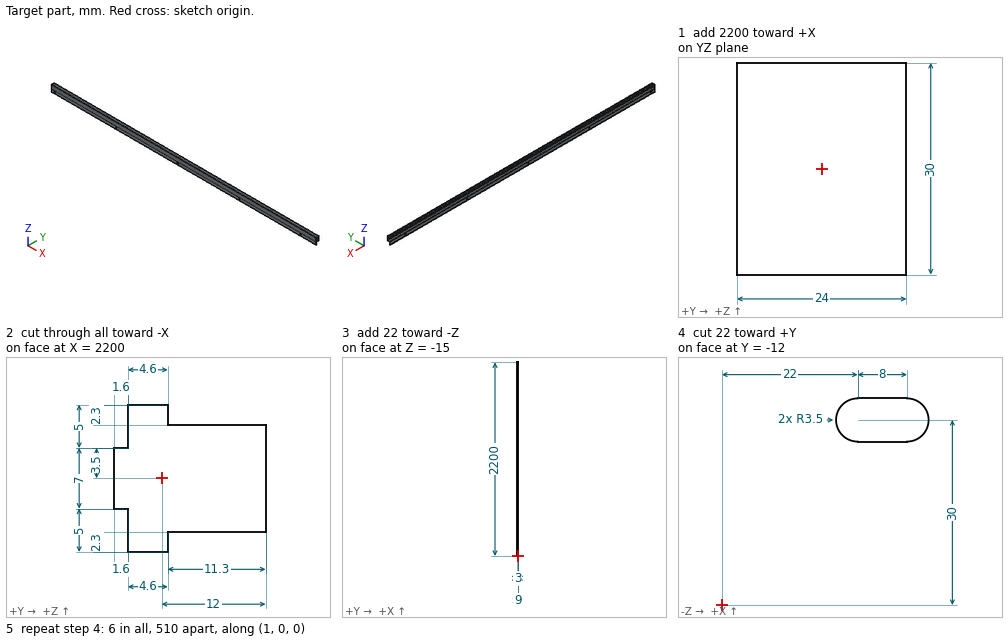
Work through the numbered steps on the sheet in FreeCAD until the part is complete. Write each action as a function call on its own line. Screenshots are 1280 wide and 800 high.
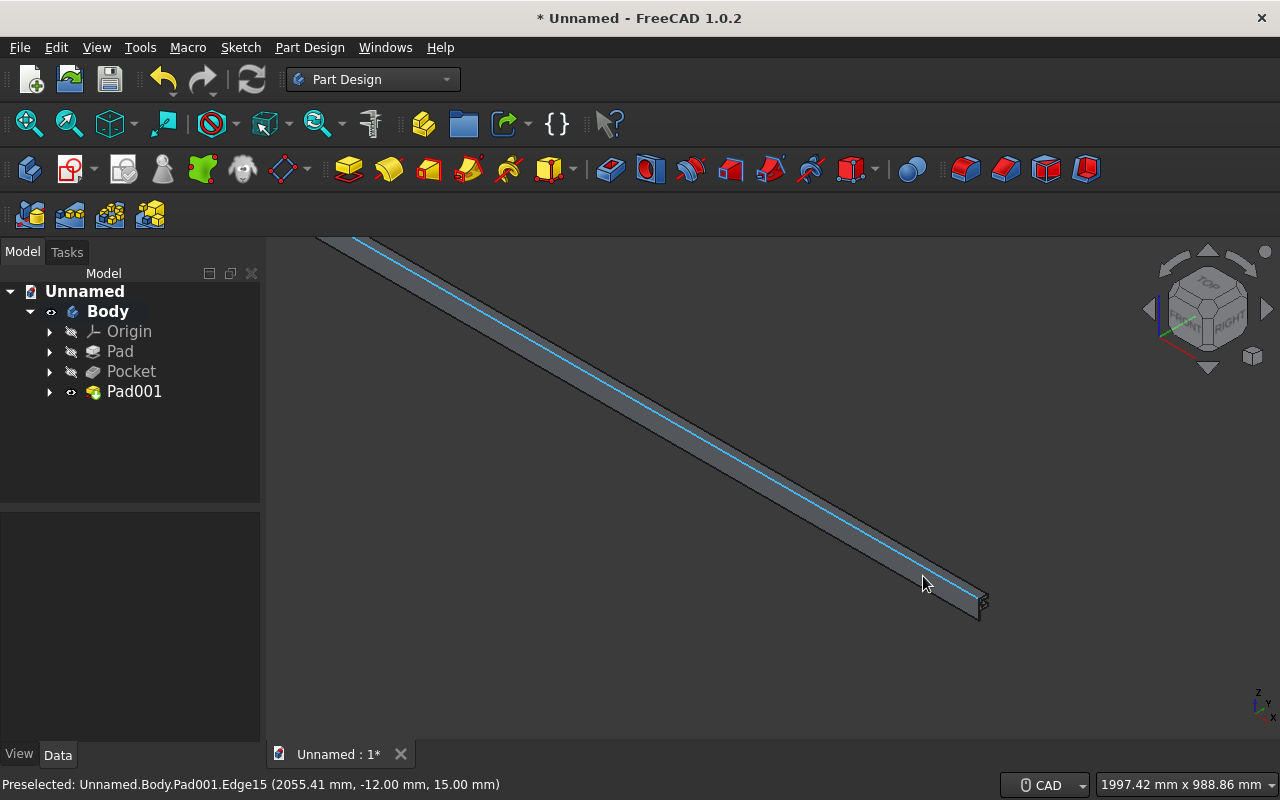
key(v)
key(f)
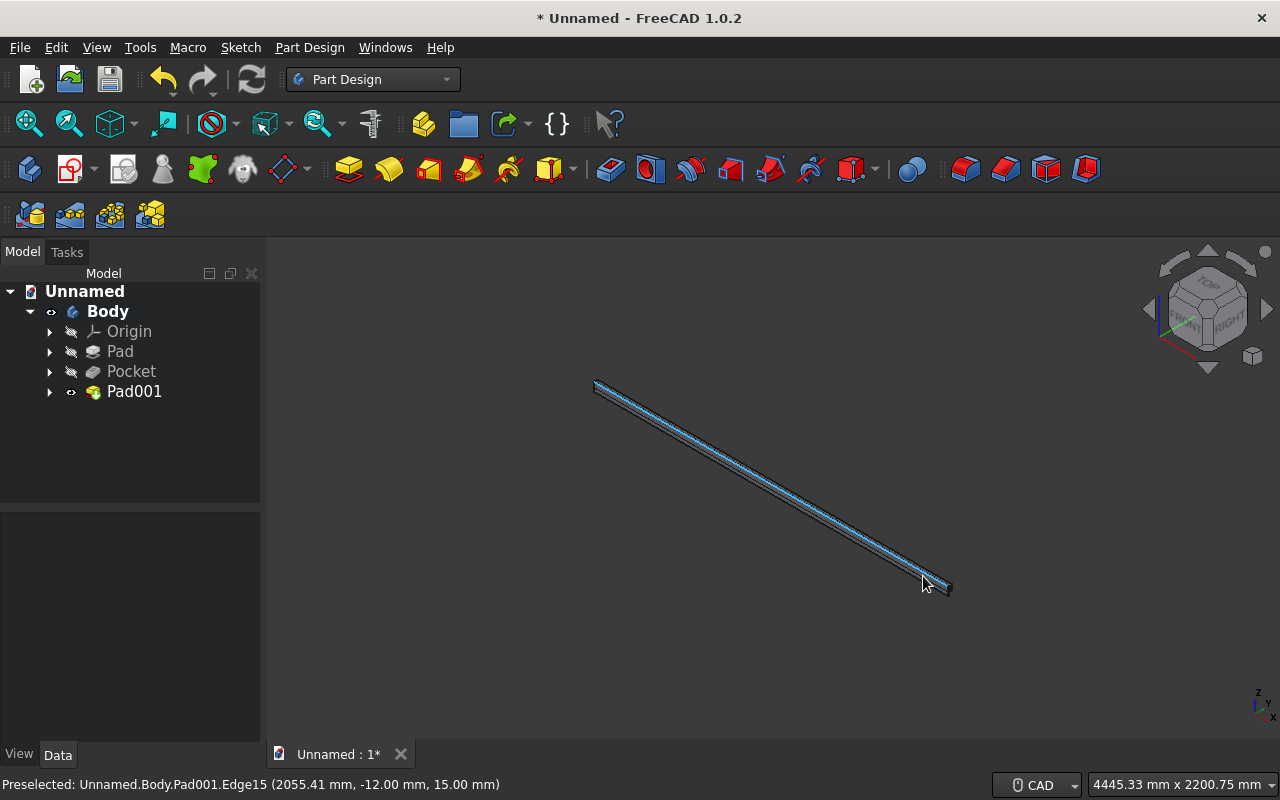
key(1)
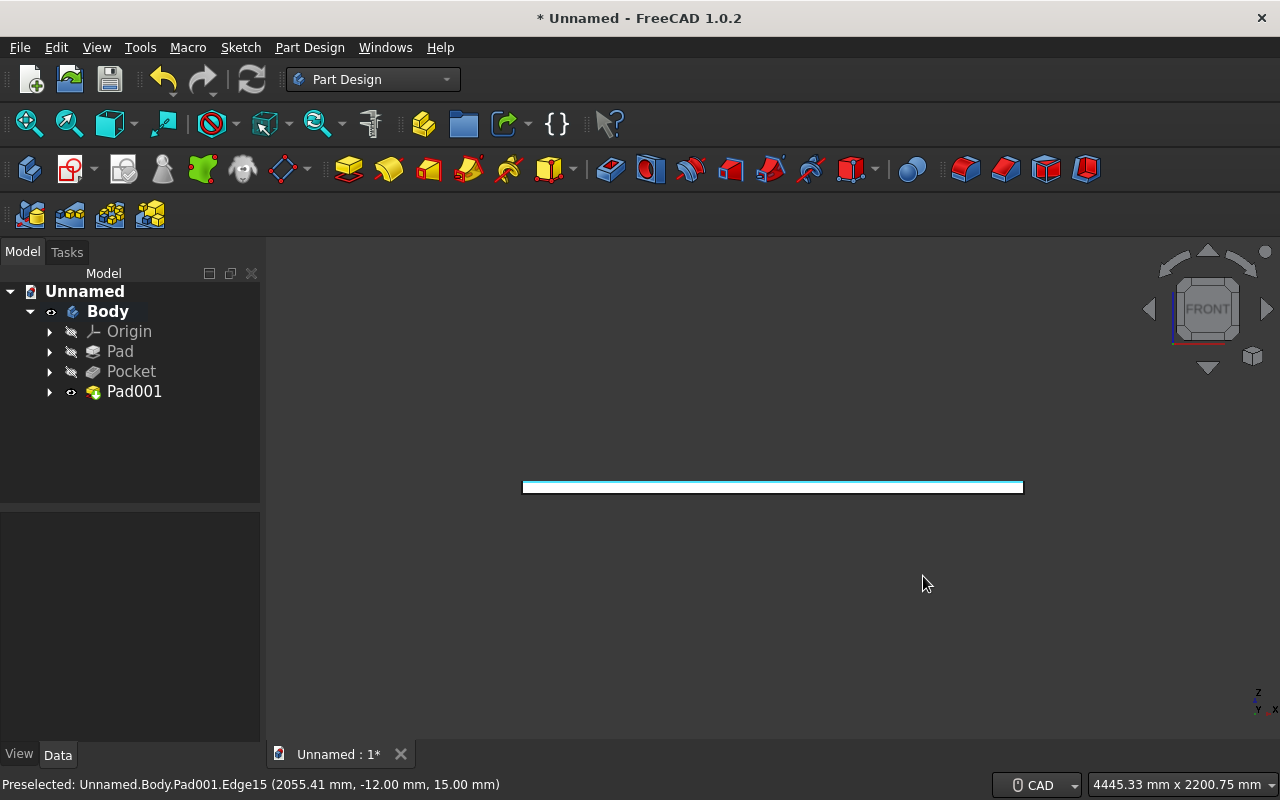
scroll(988, 487, up, 4)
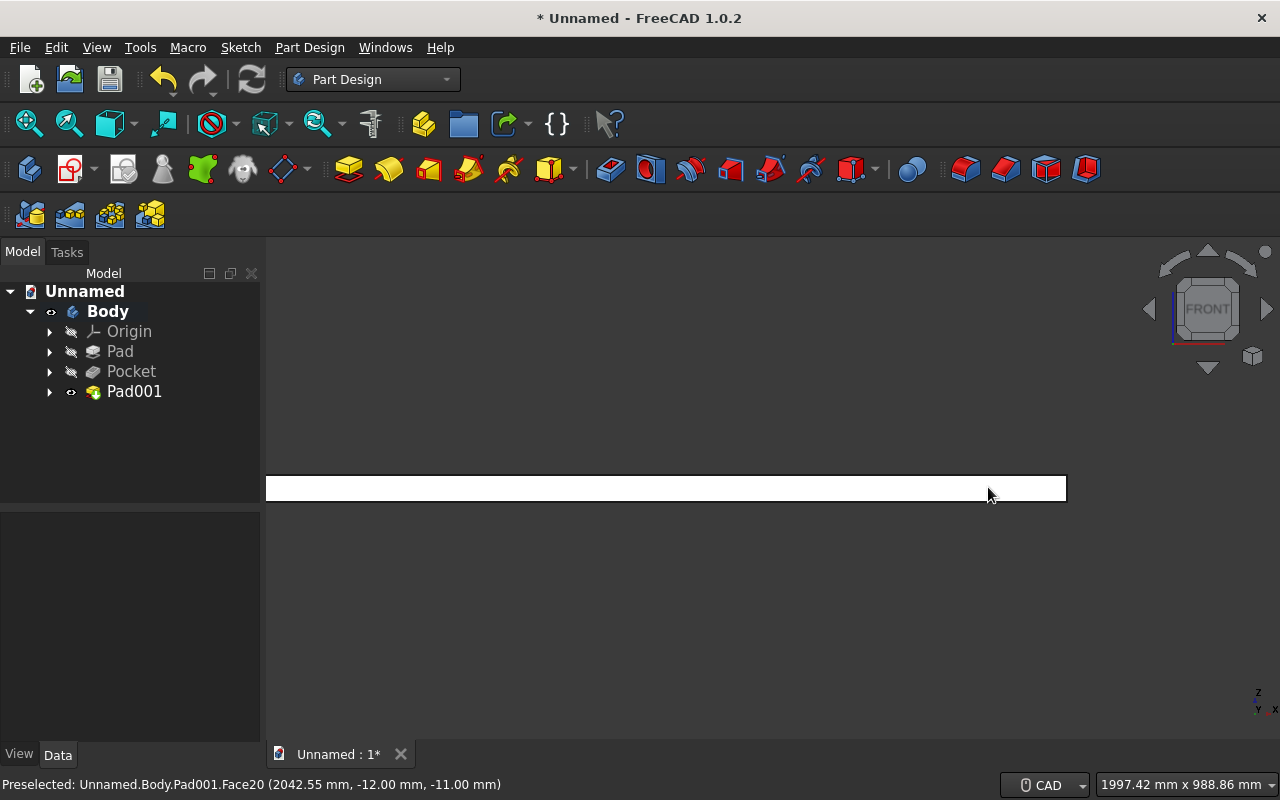
click(987, 488)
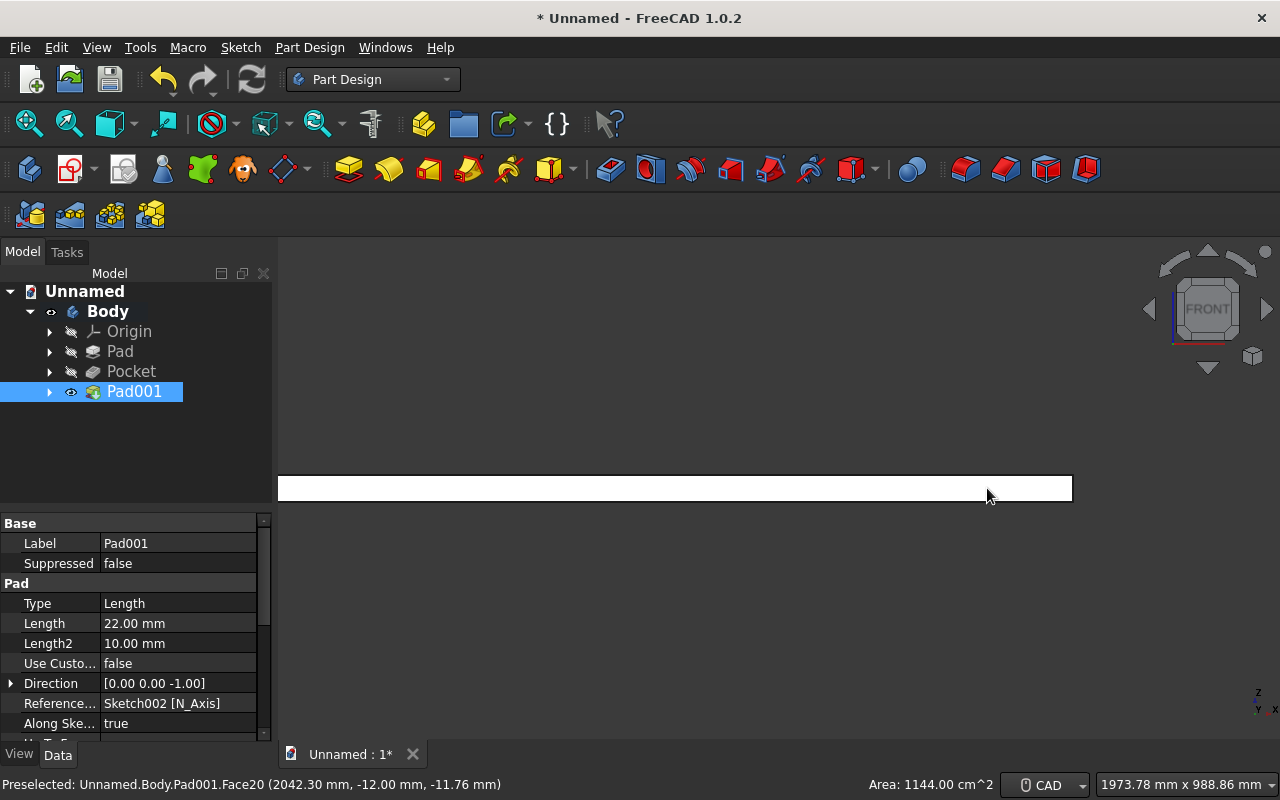
click(70, 170)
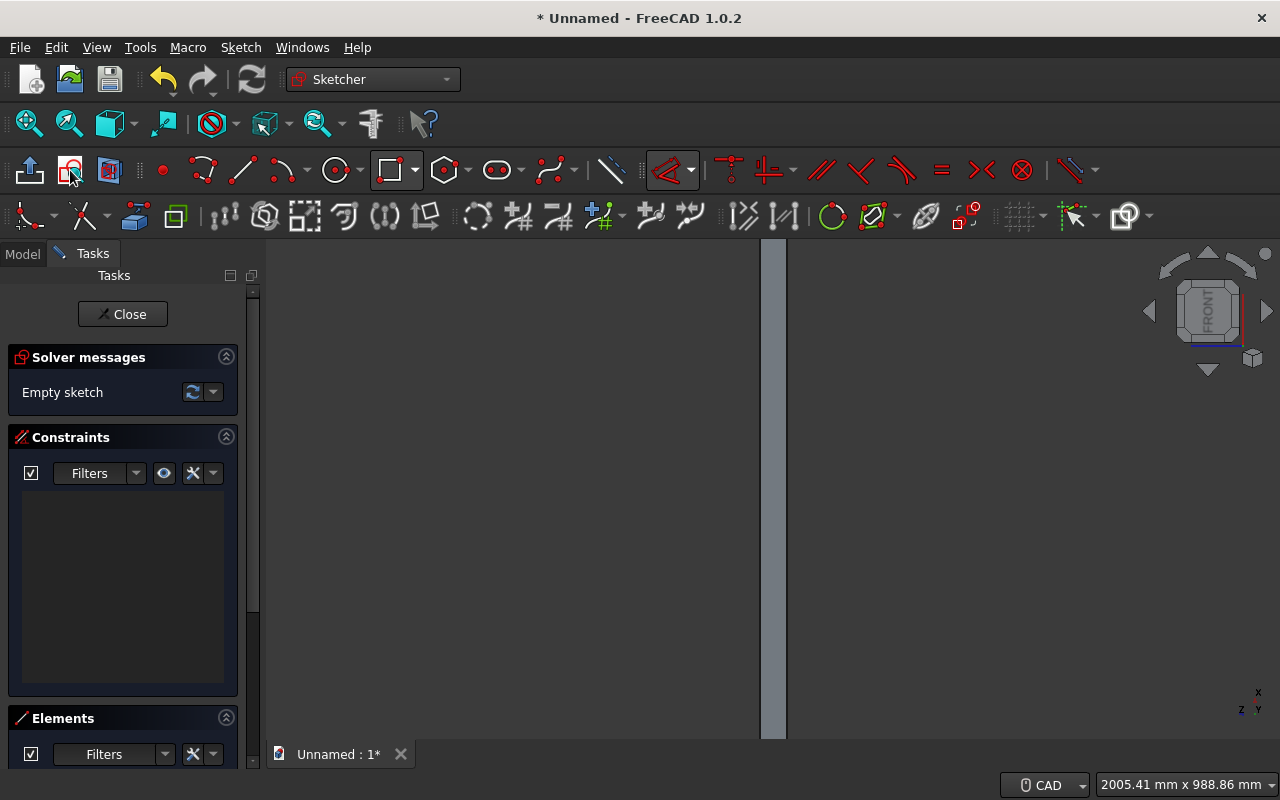
scroll(704, 489, down, 5)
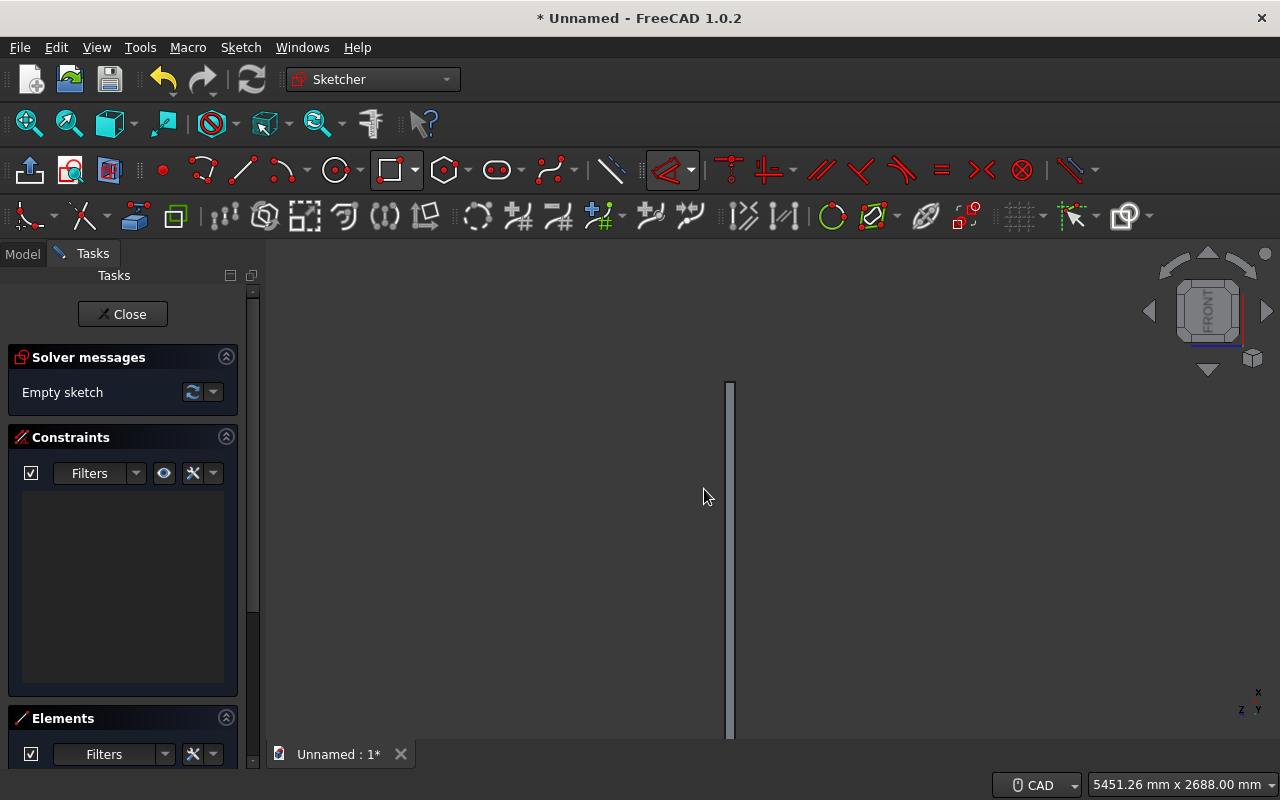
scroll(704, 489, down, 5)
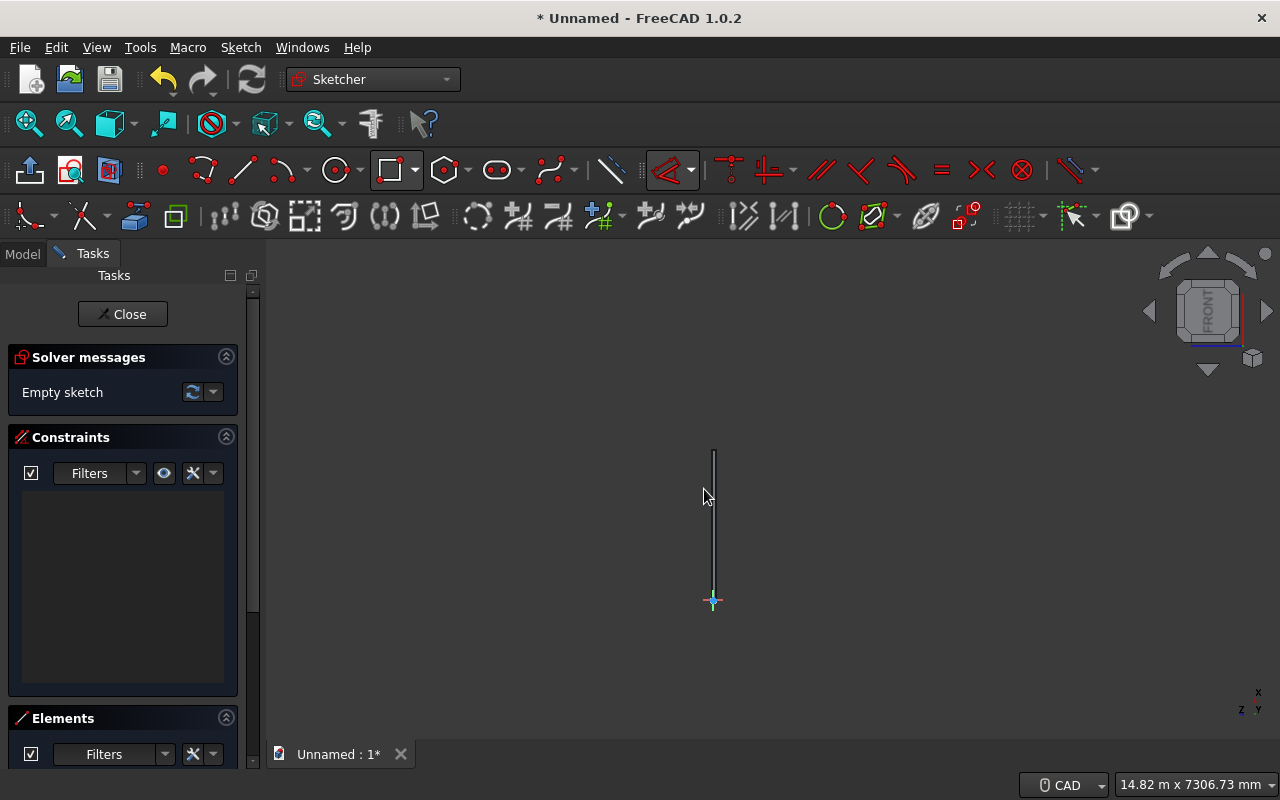
scroll(715, 605, up, 15)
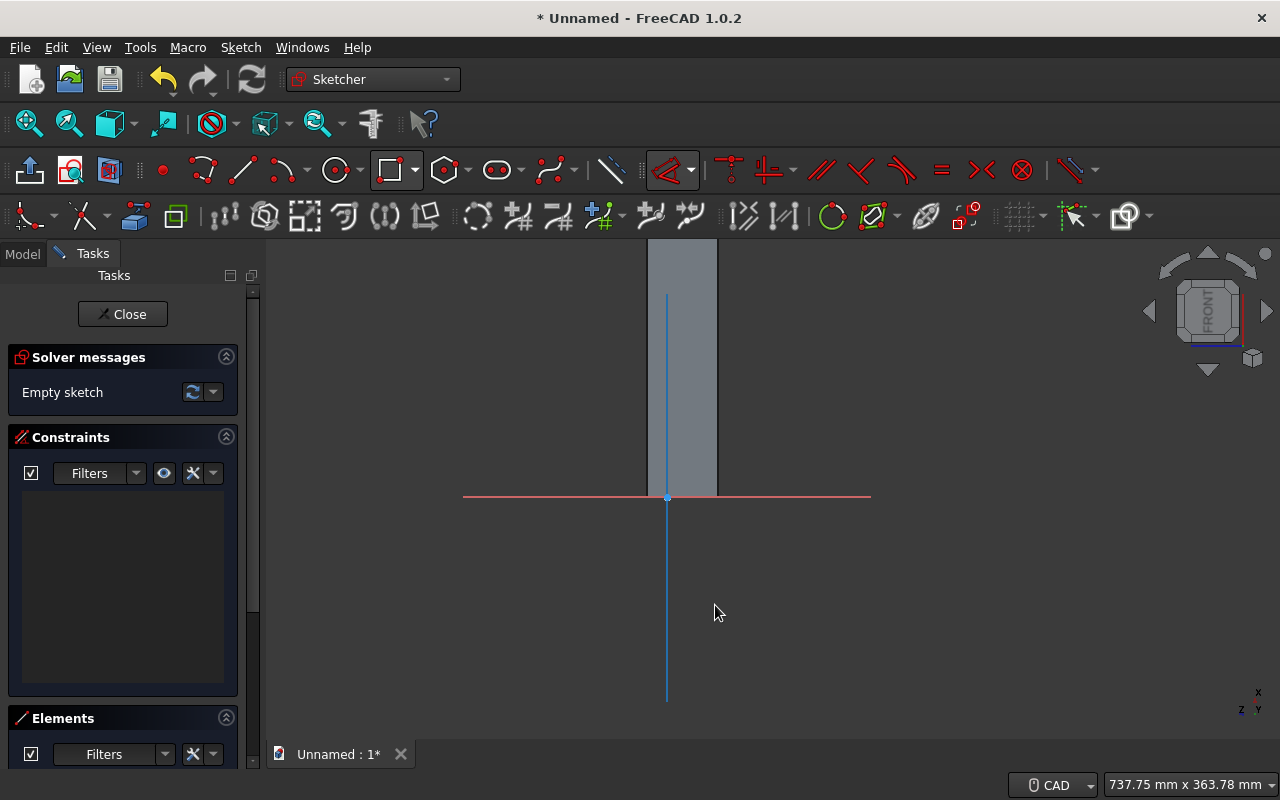
scroll(688, 472, up, 10)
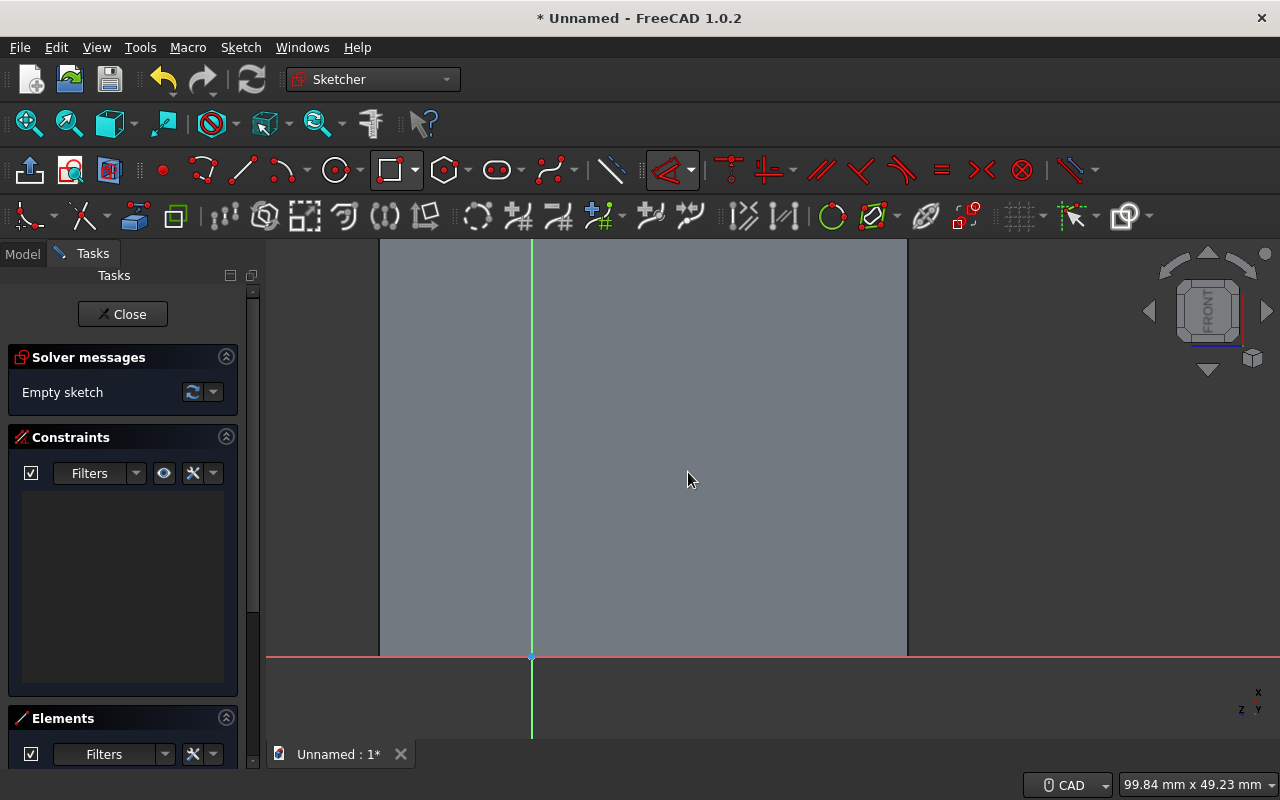
click(498, 170)